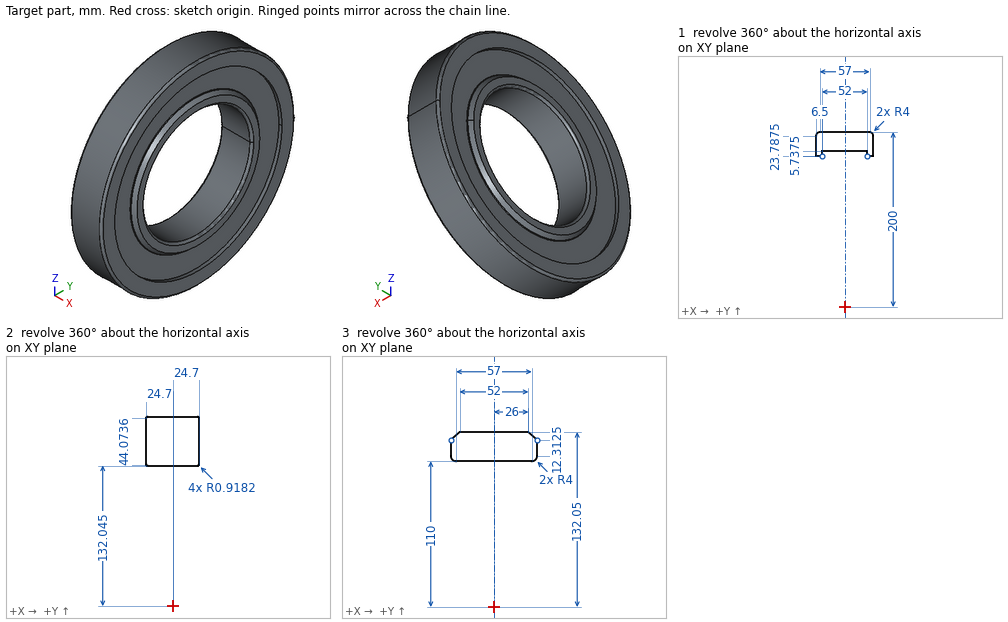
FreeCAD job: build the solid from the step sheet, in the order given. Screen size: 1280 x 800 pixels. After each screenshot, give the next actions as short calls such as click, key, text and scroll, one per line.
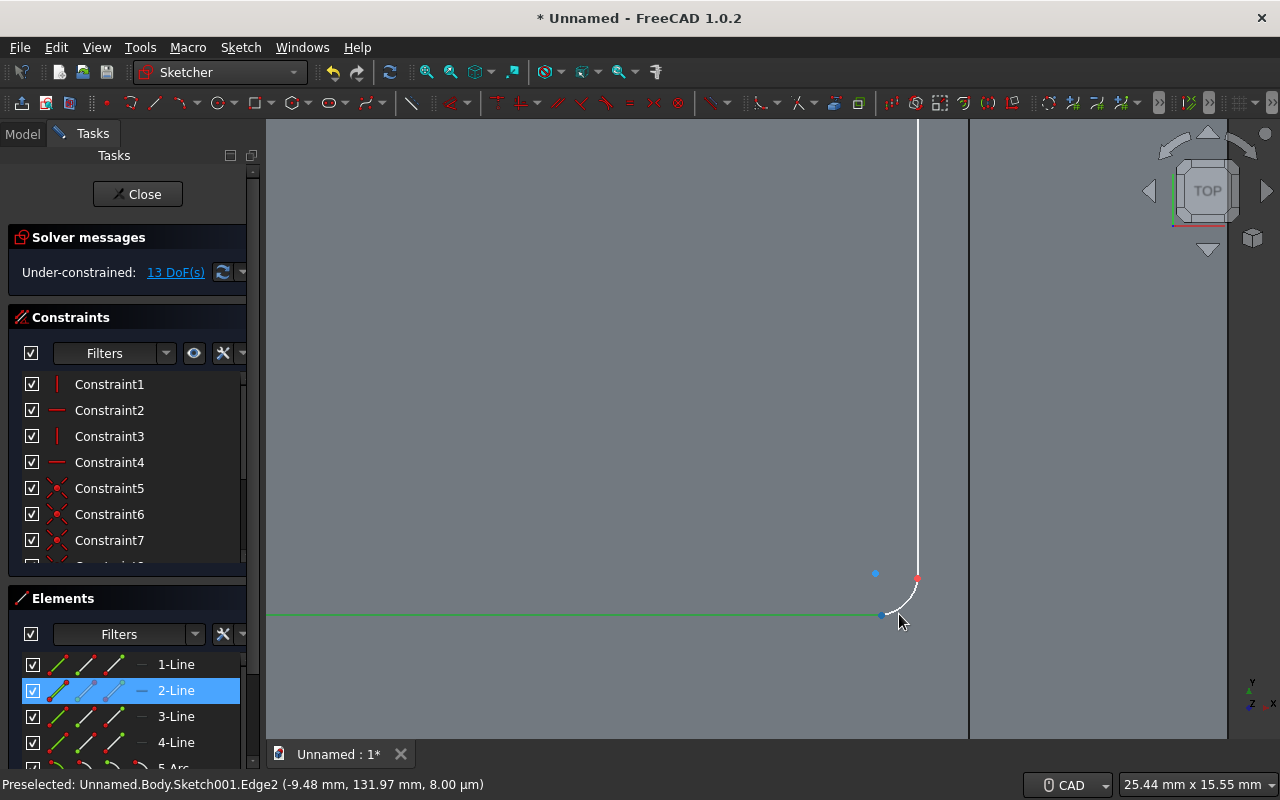
click(897, 610)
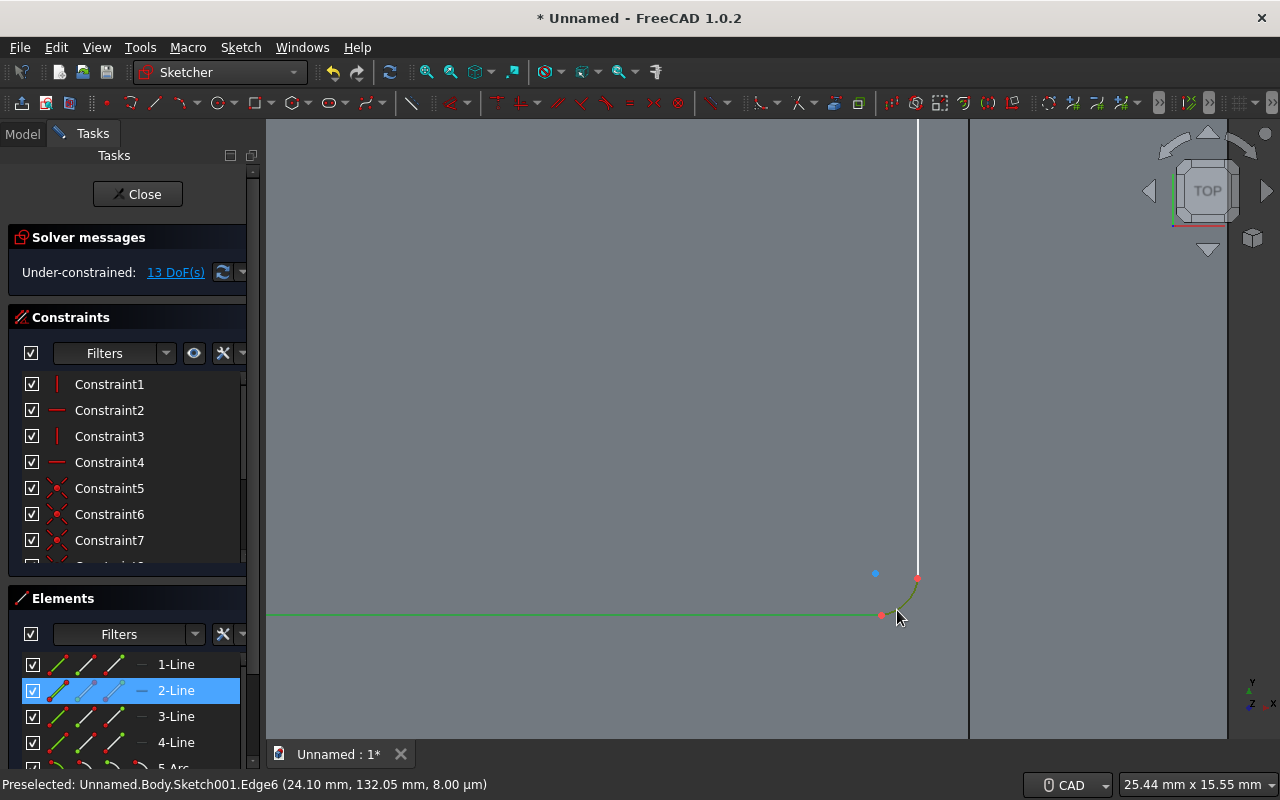
click(606, 104)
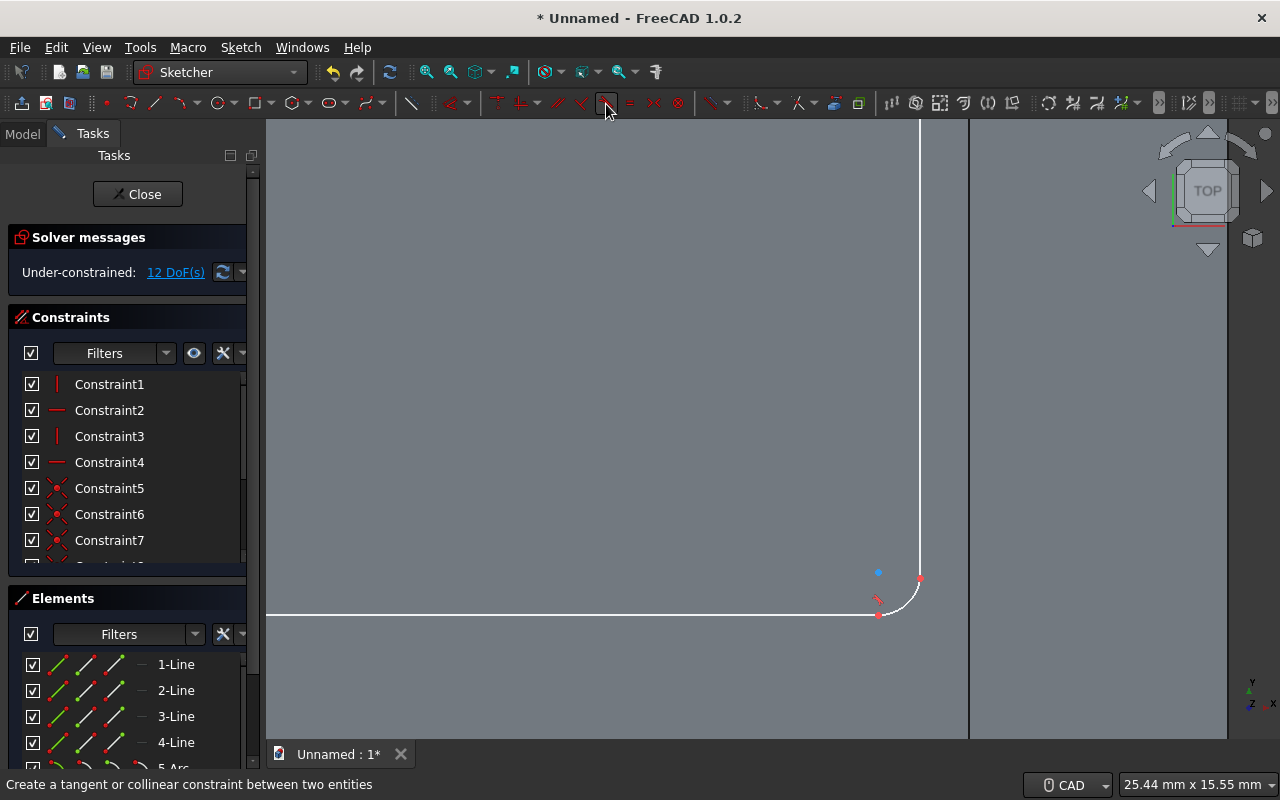
scroll(900, 614, down, 8)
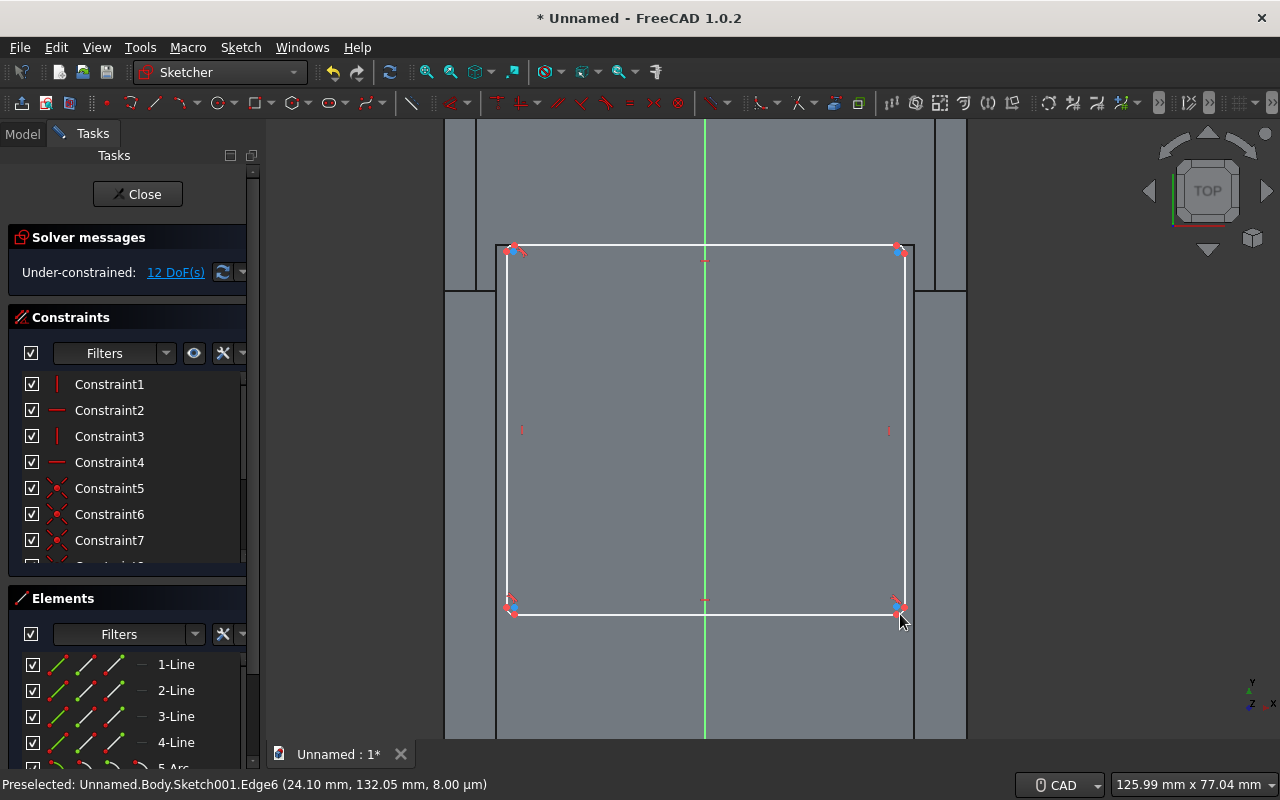
click(905, 537)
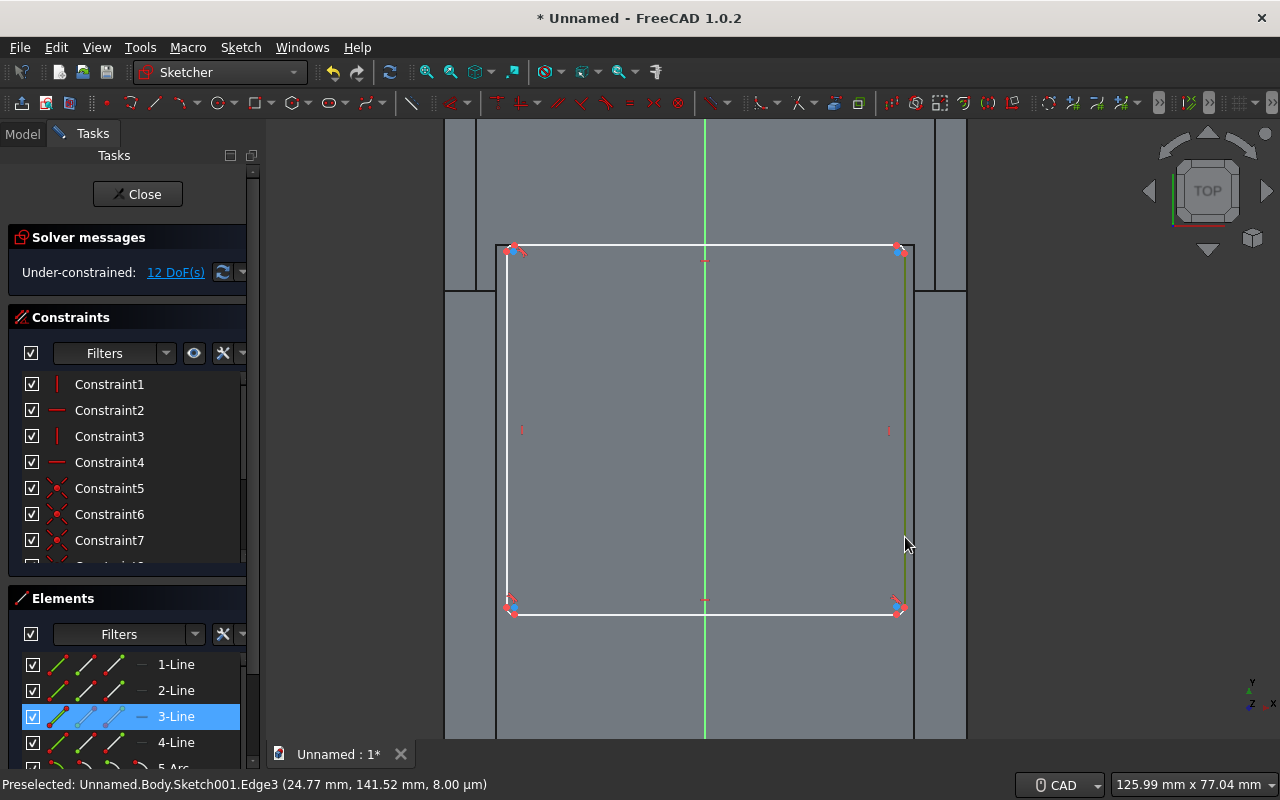
scroll(902, 613, up, 5)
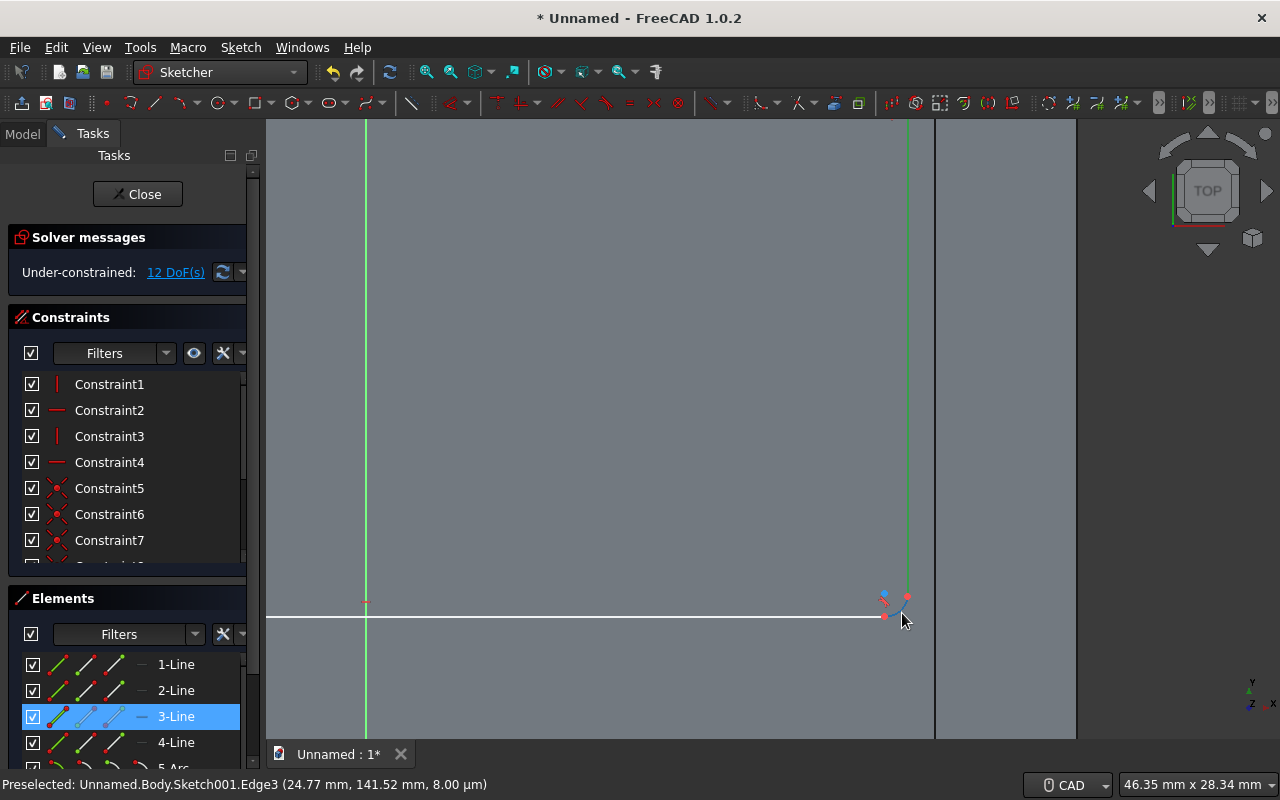
click(900, 611)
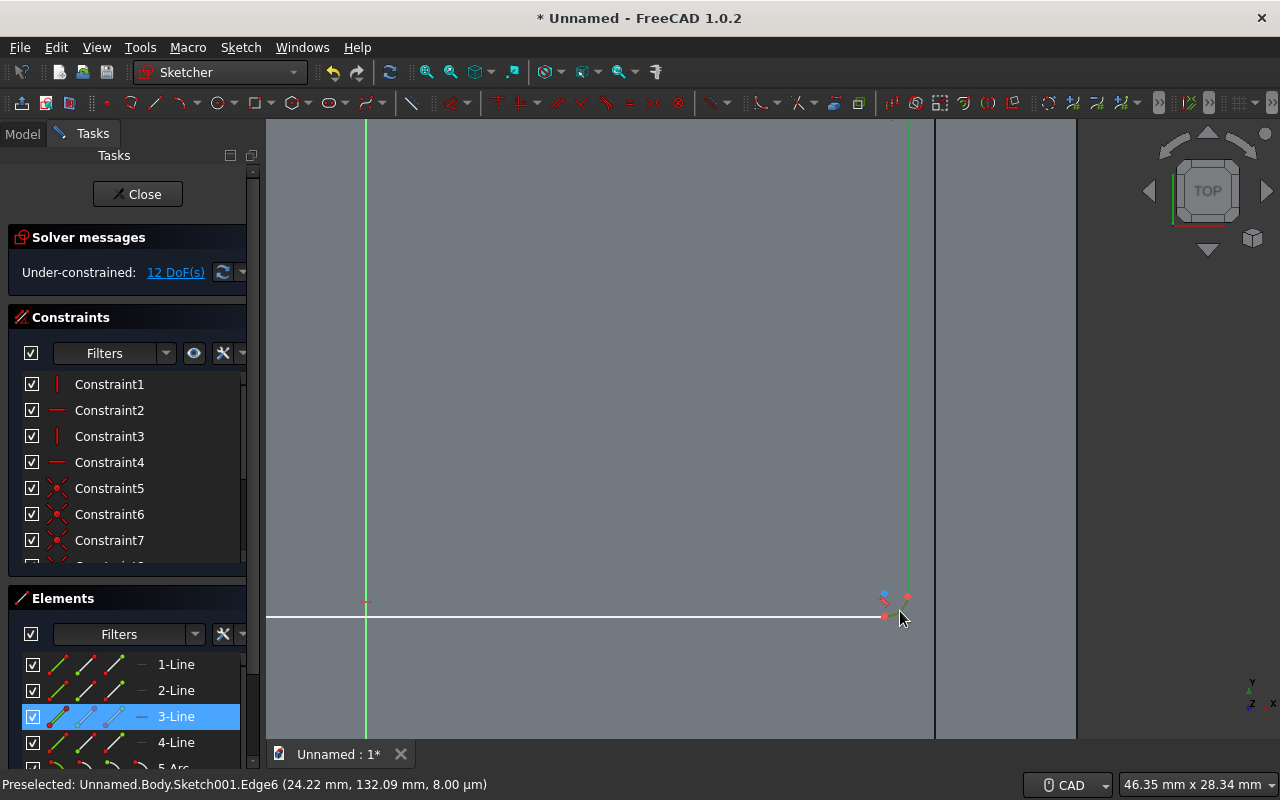
click(606, 104)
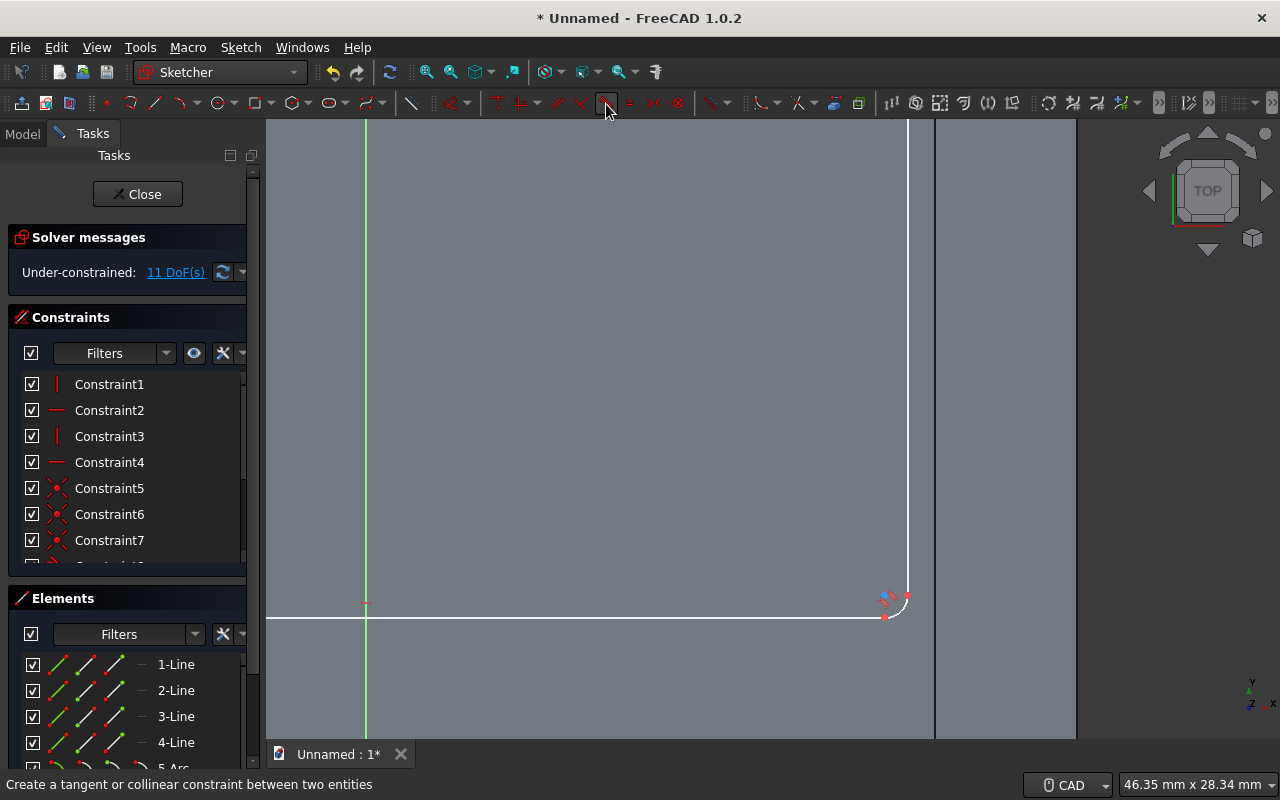
click(908, 307)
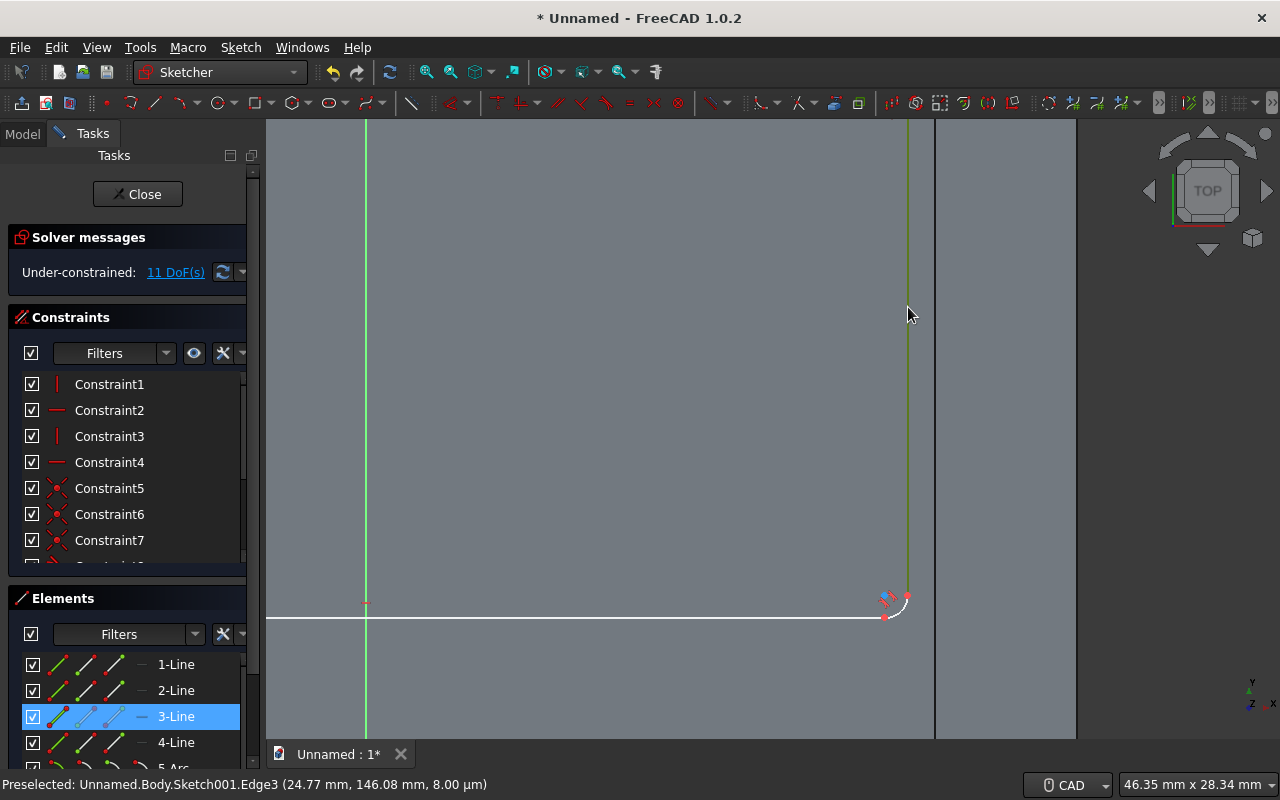
scroll(902, 613, down, 5)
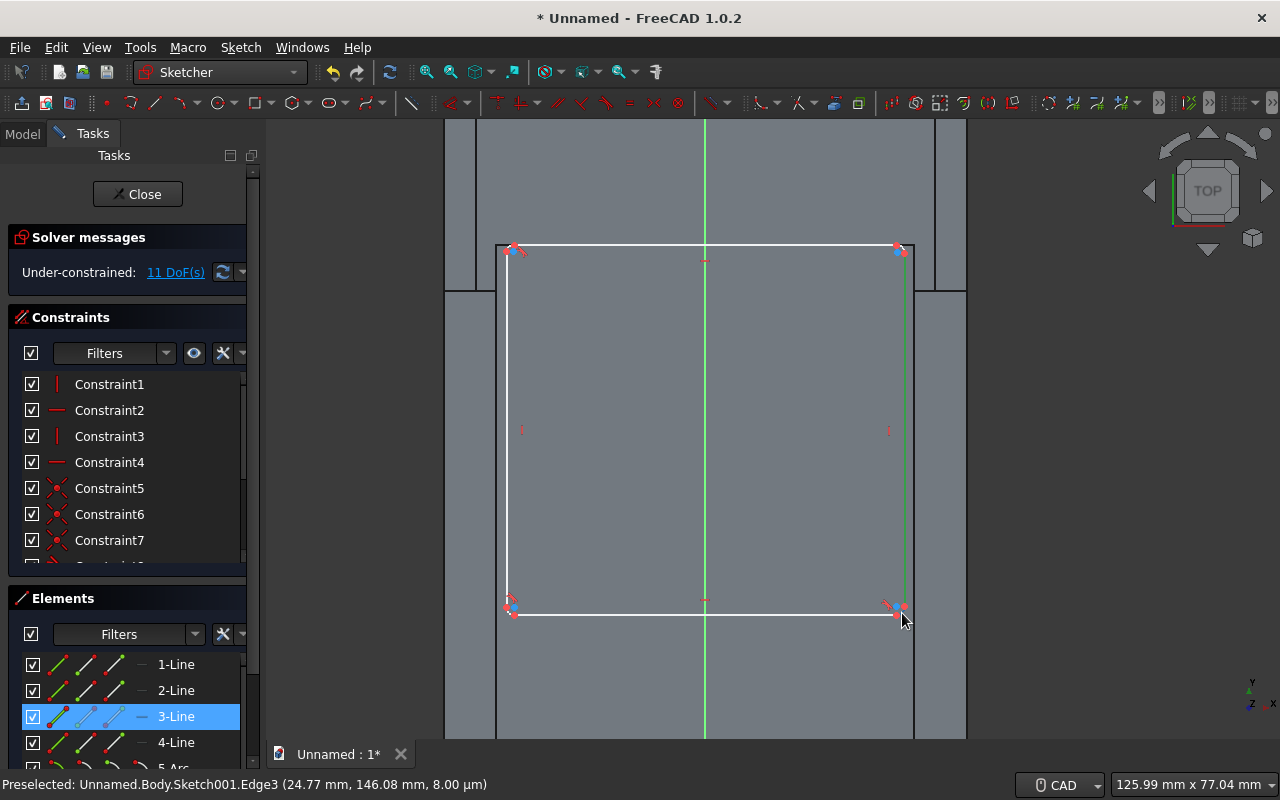
scroll(904, 250, up, 7)